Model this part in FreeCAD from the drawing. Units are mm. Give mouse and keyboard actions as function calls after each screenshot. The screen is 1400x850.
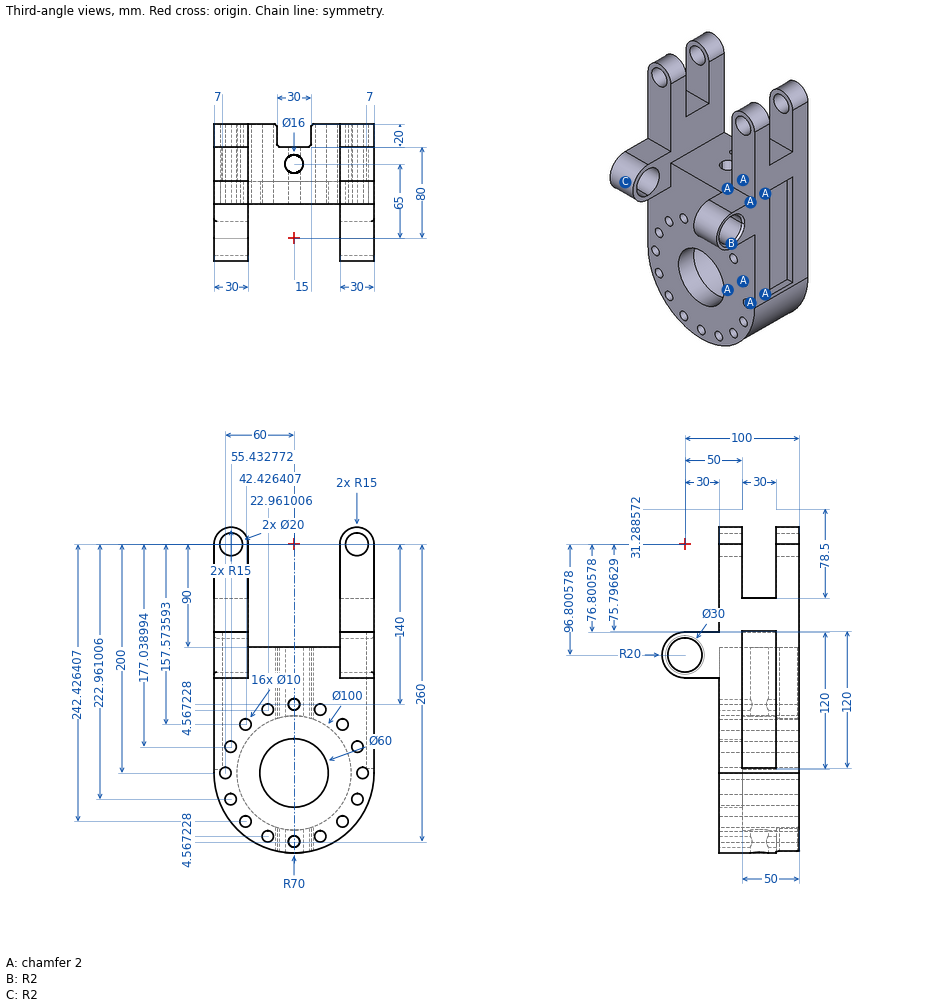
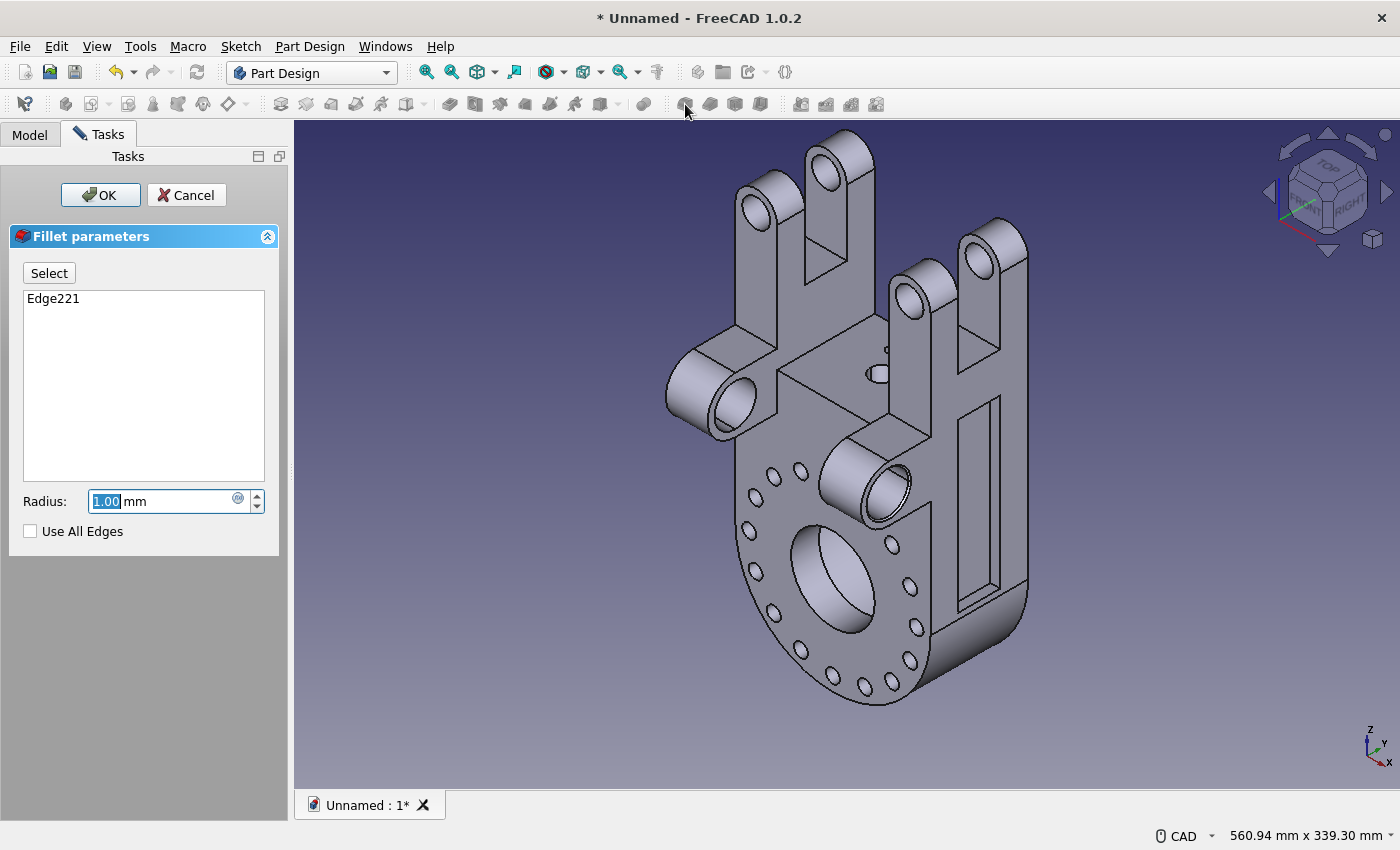
text(2)
key(Tab)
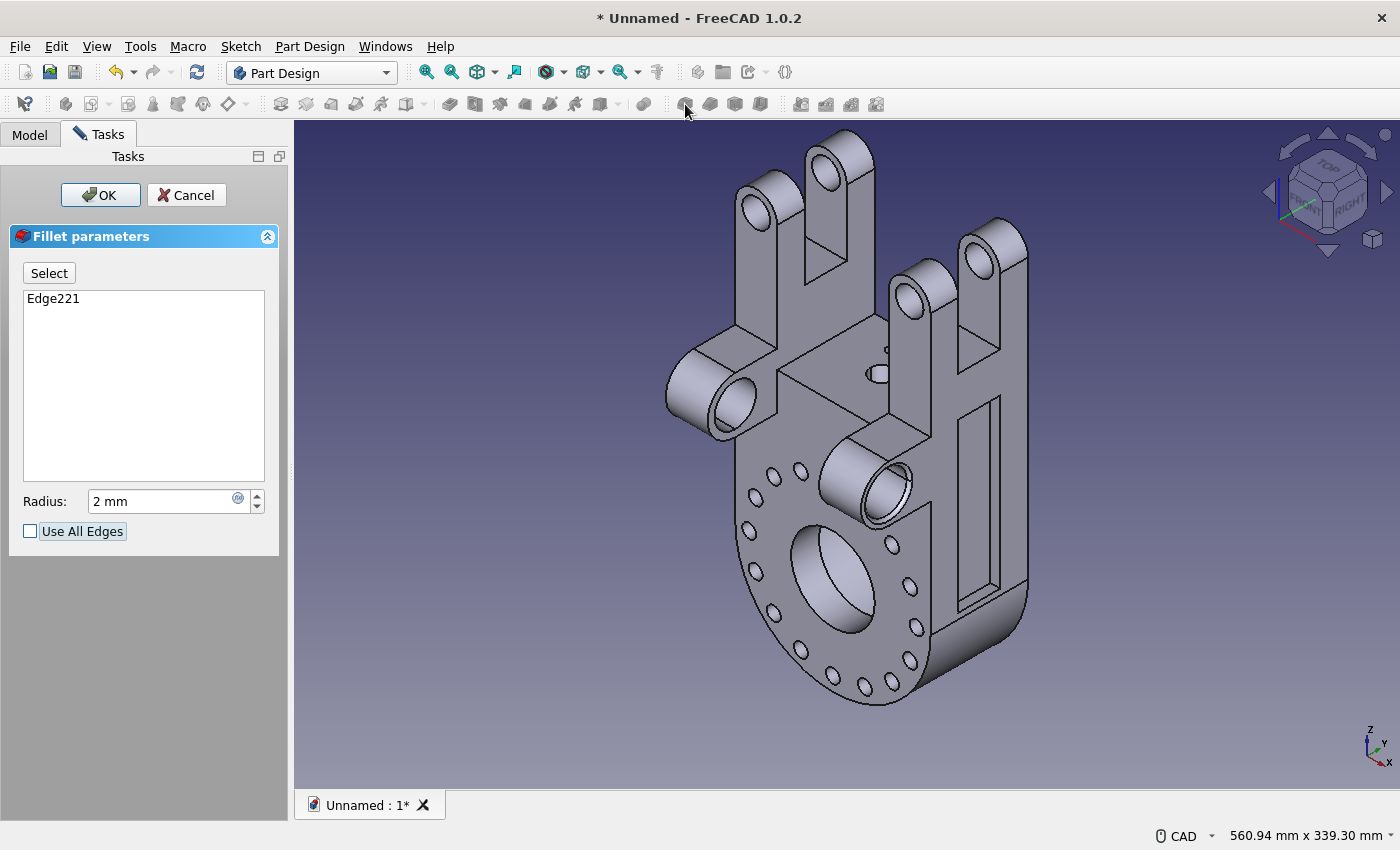
click(101, 195)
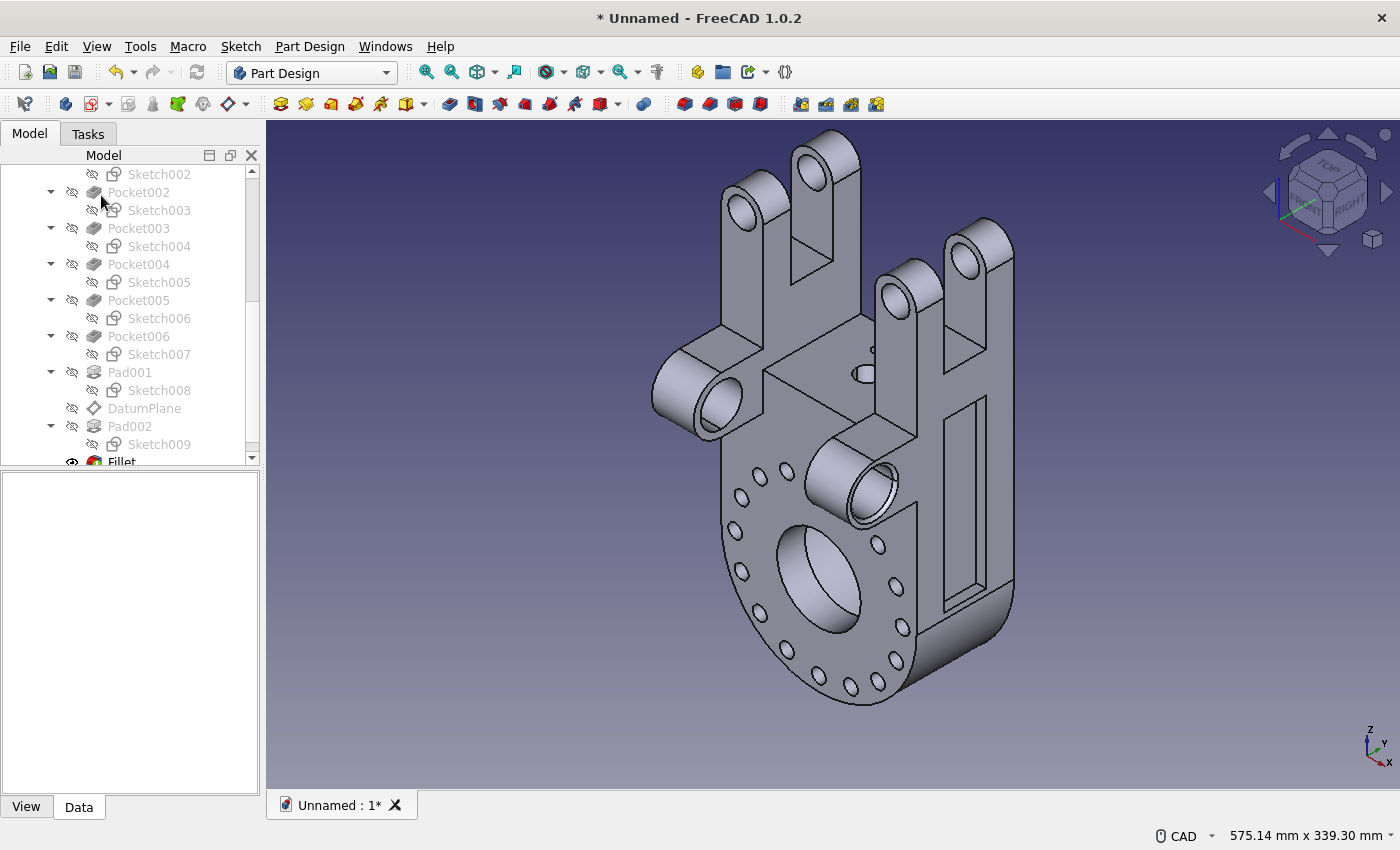
click(427, 72)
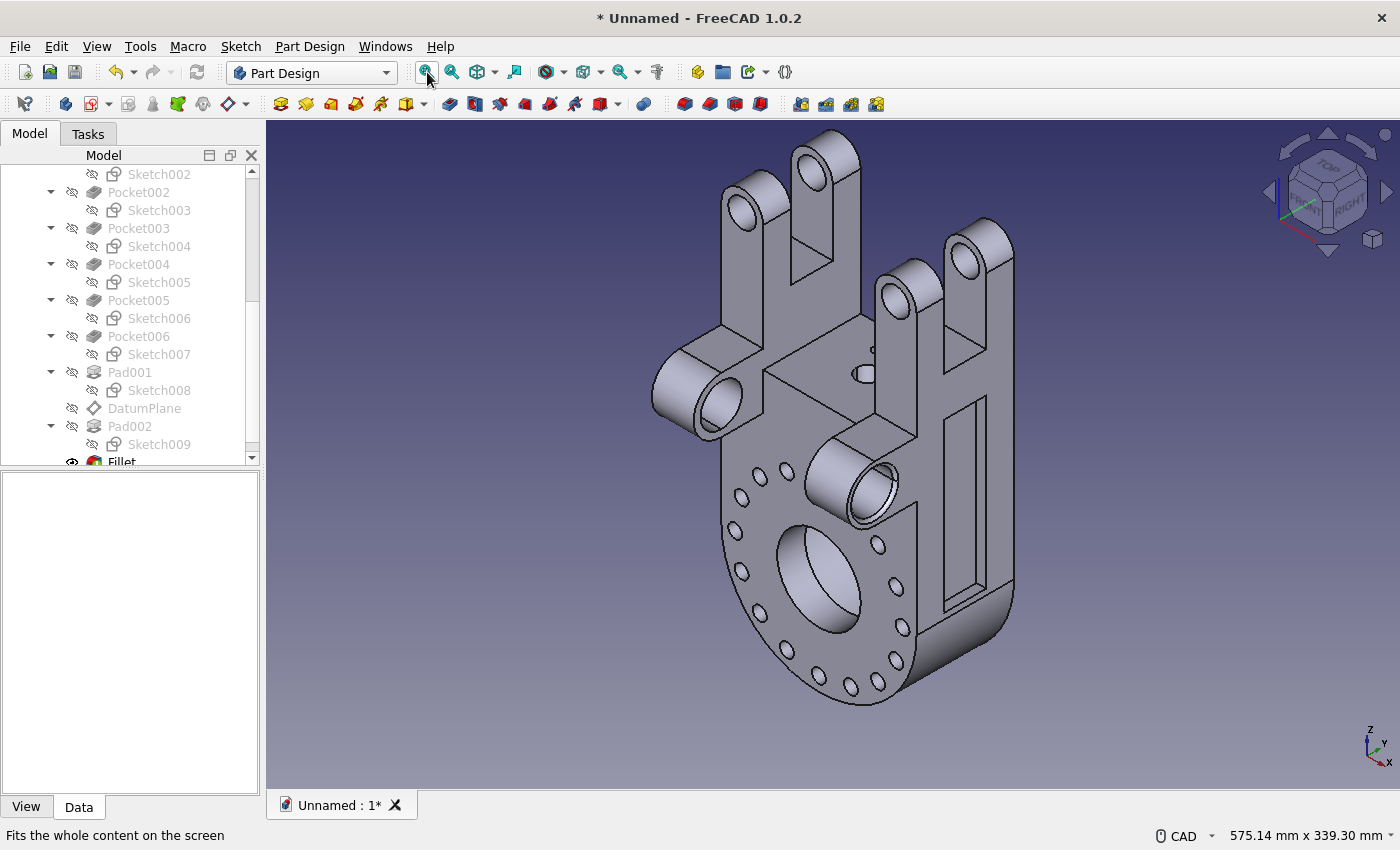
key(2)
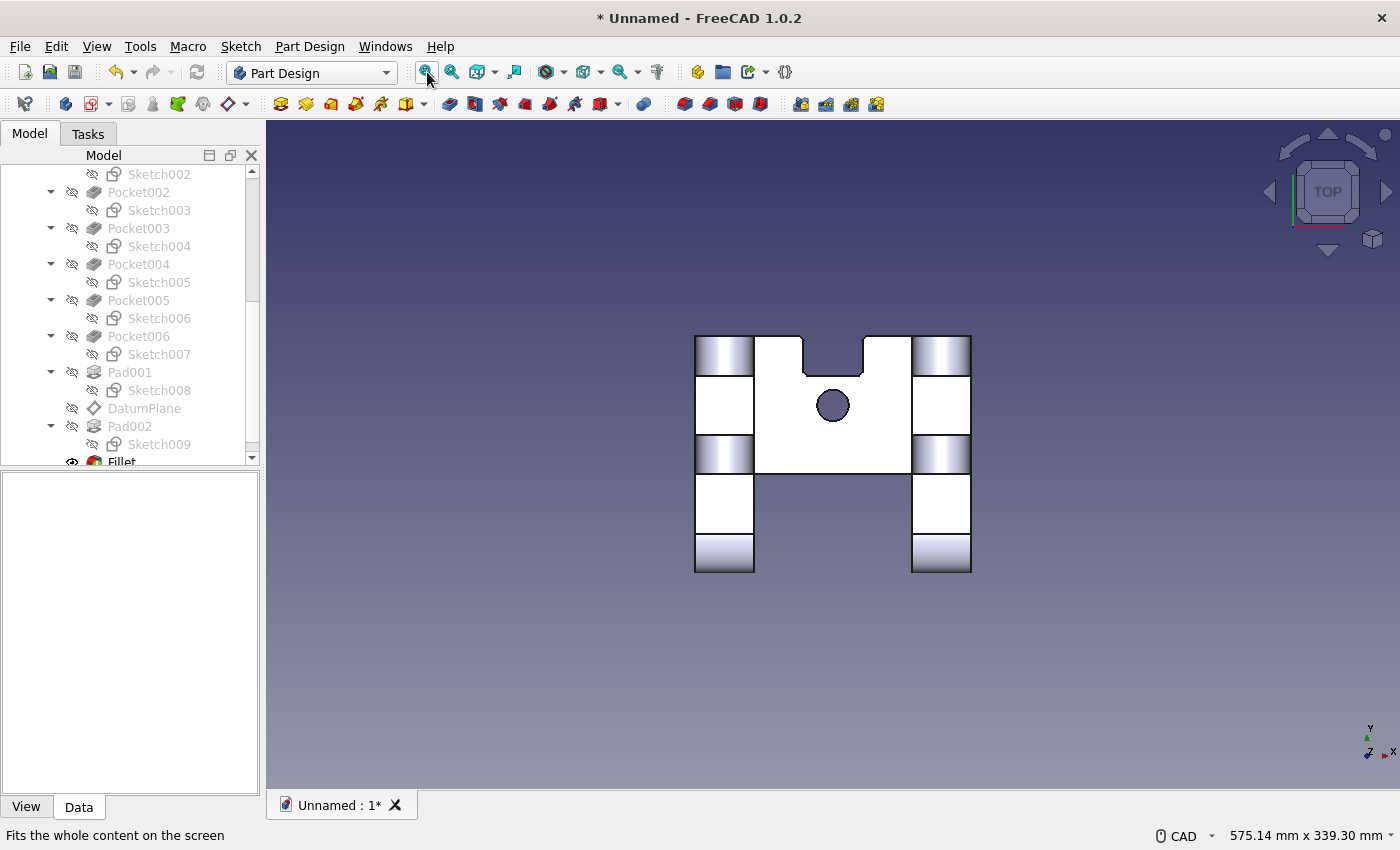
key(v)
key(f)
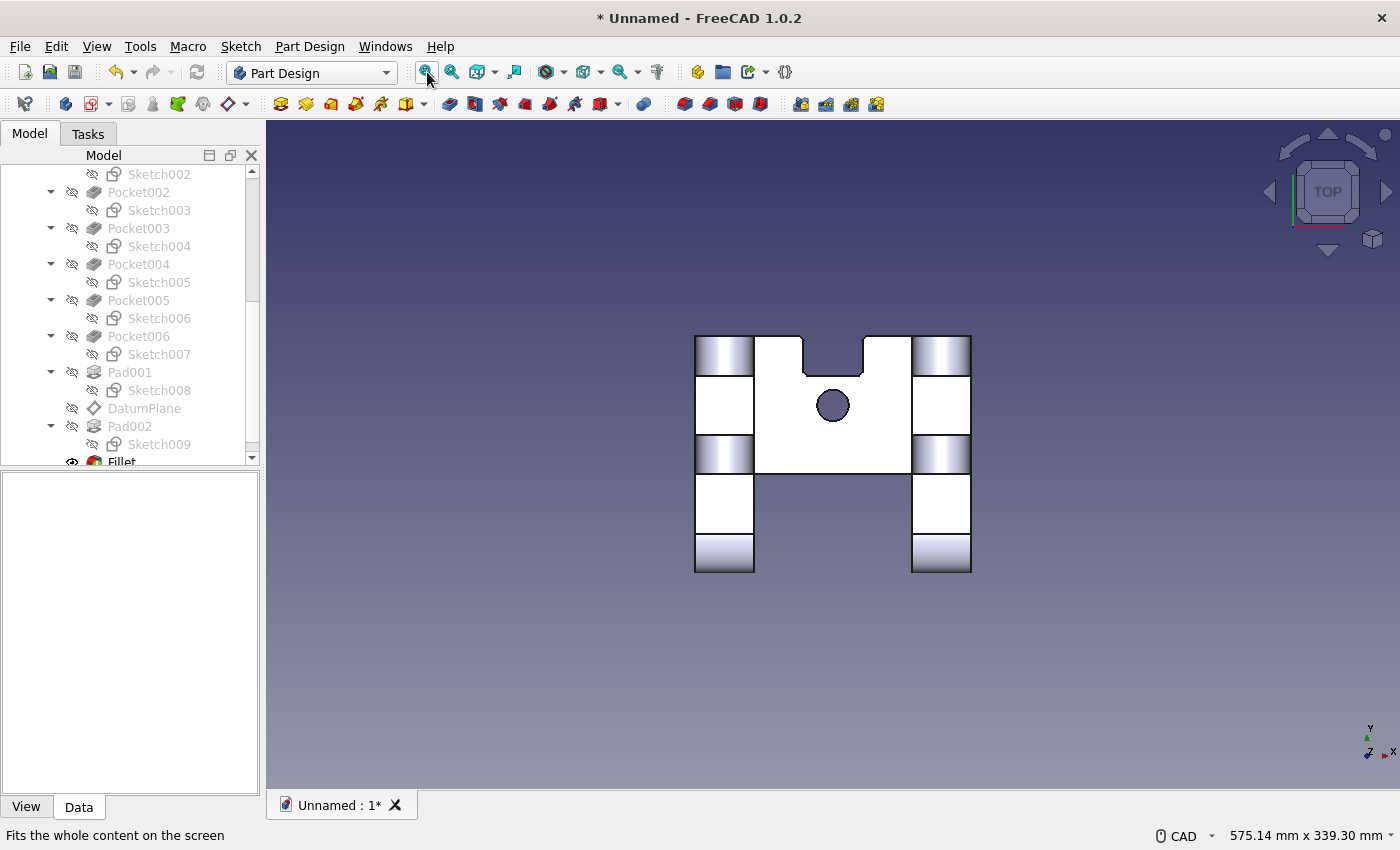
key(0)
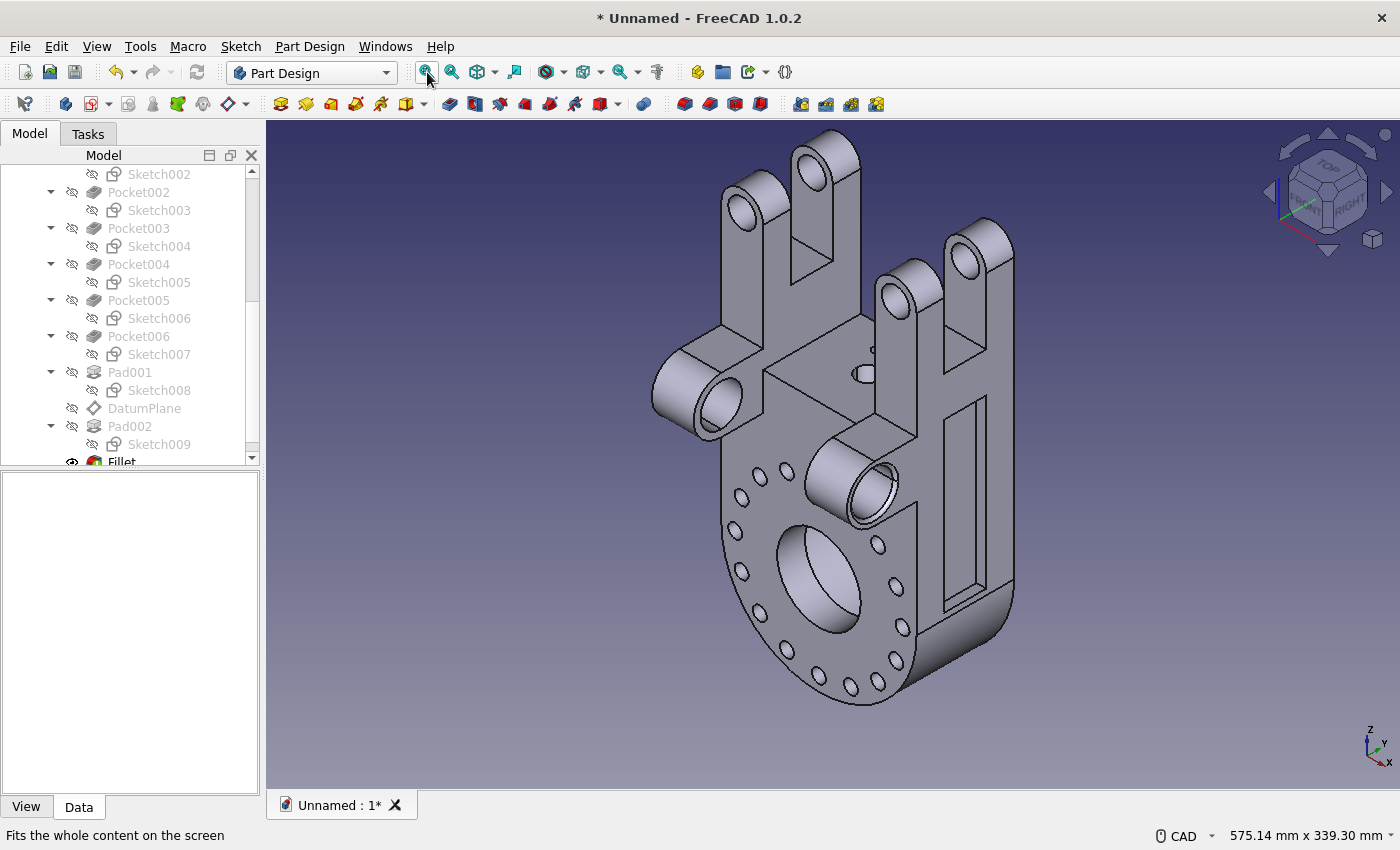
click(427, 72)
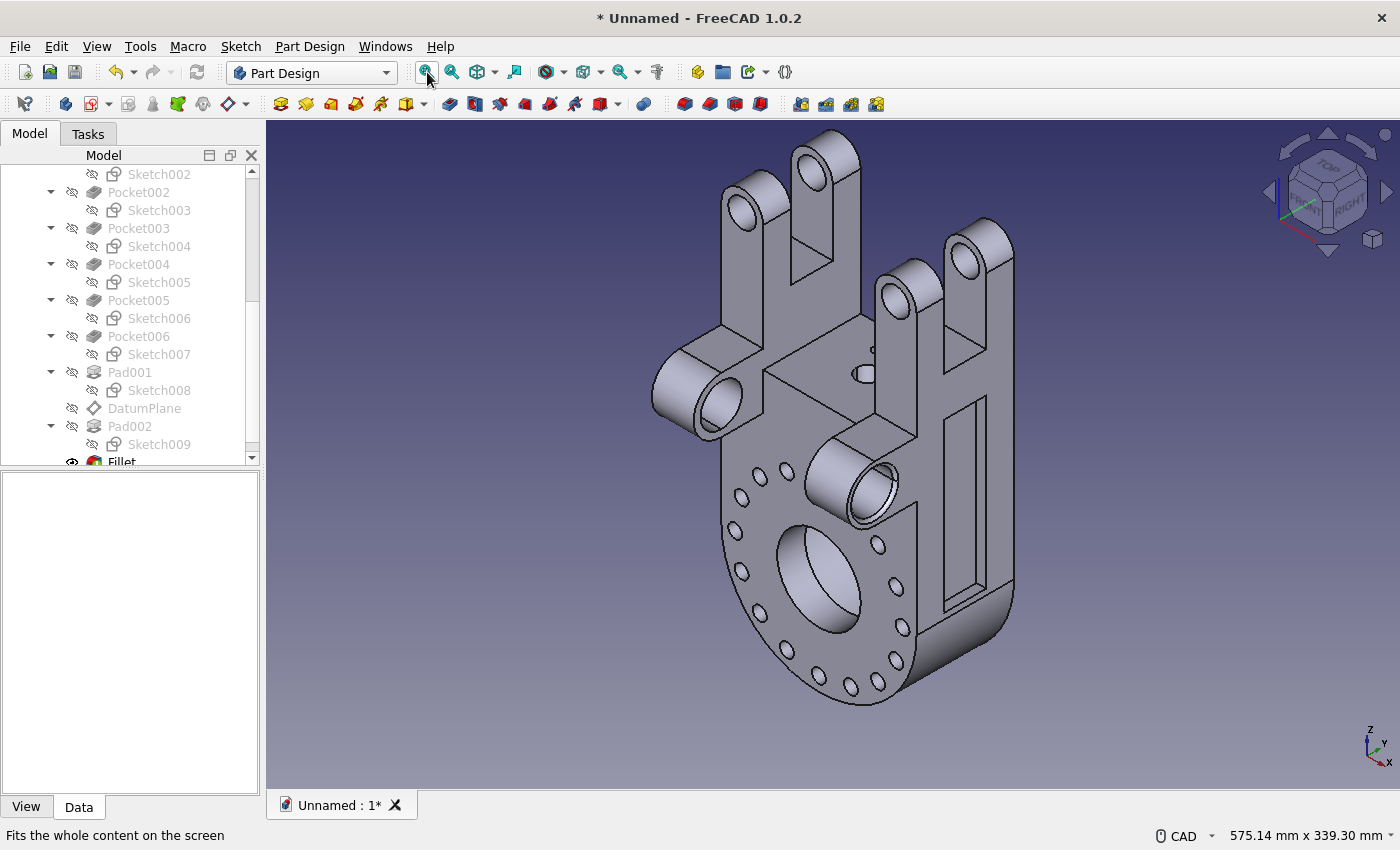
key(1)